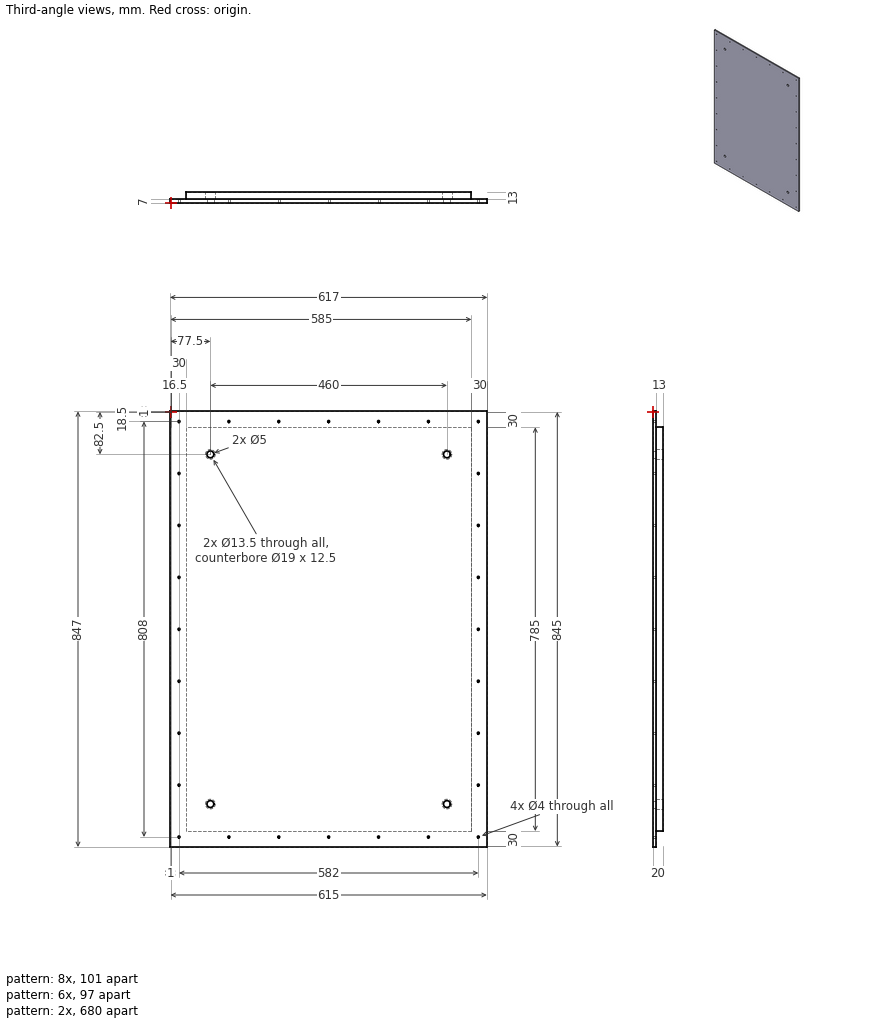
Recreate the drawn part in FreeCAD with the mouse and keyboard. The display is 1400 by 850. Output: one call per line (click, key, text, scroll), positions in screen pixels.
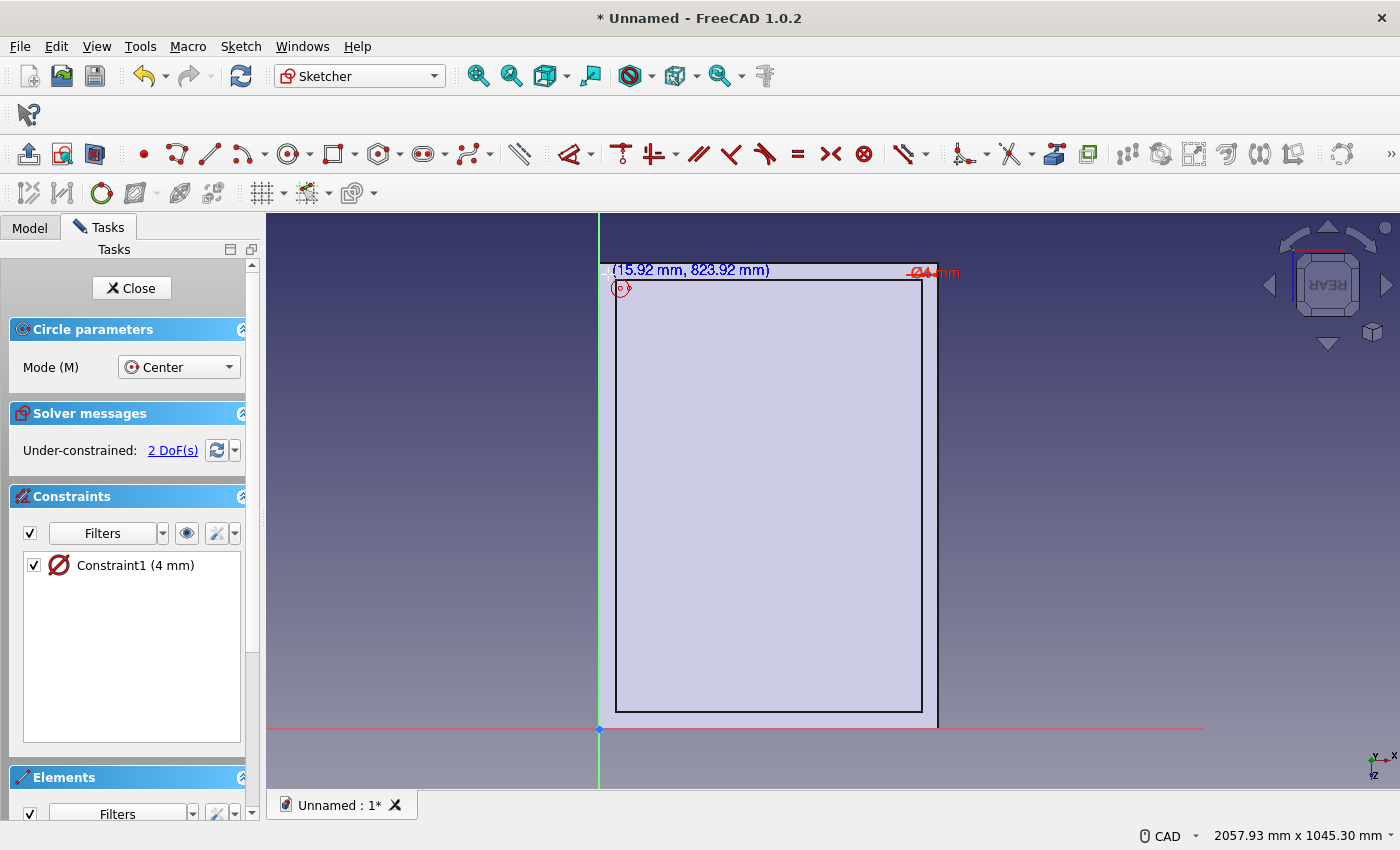
scroll(608, 274, up, 3)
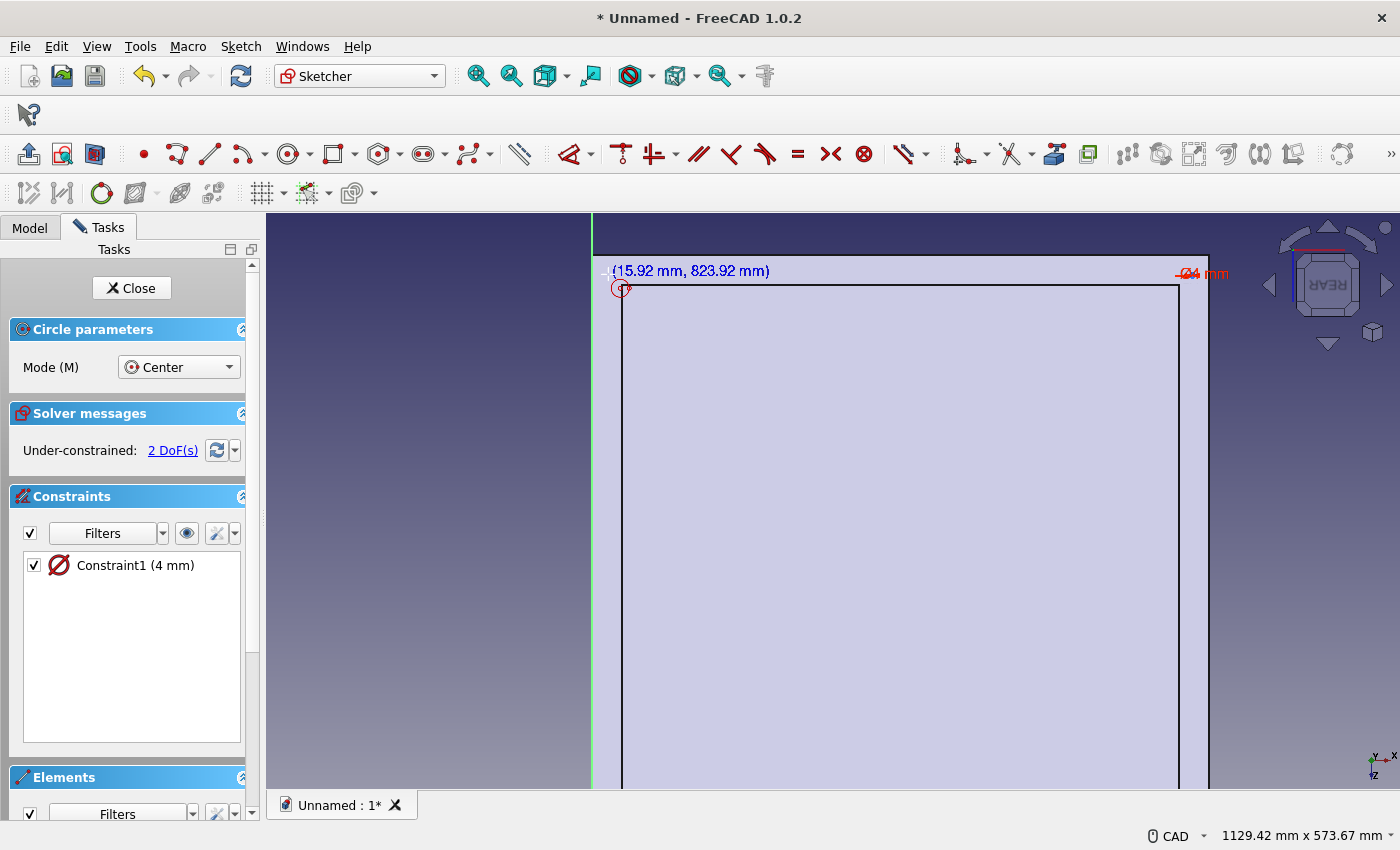
click(608, 273)
move(610, 272)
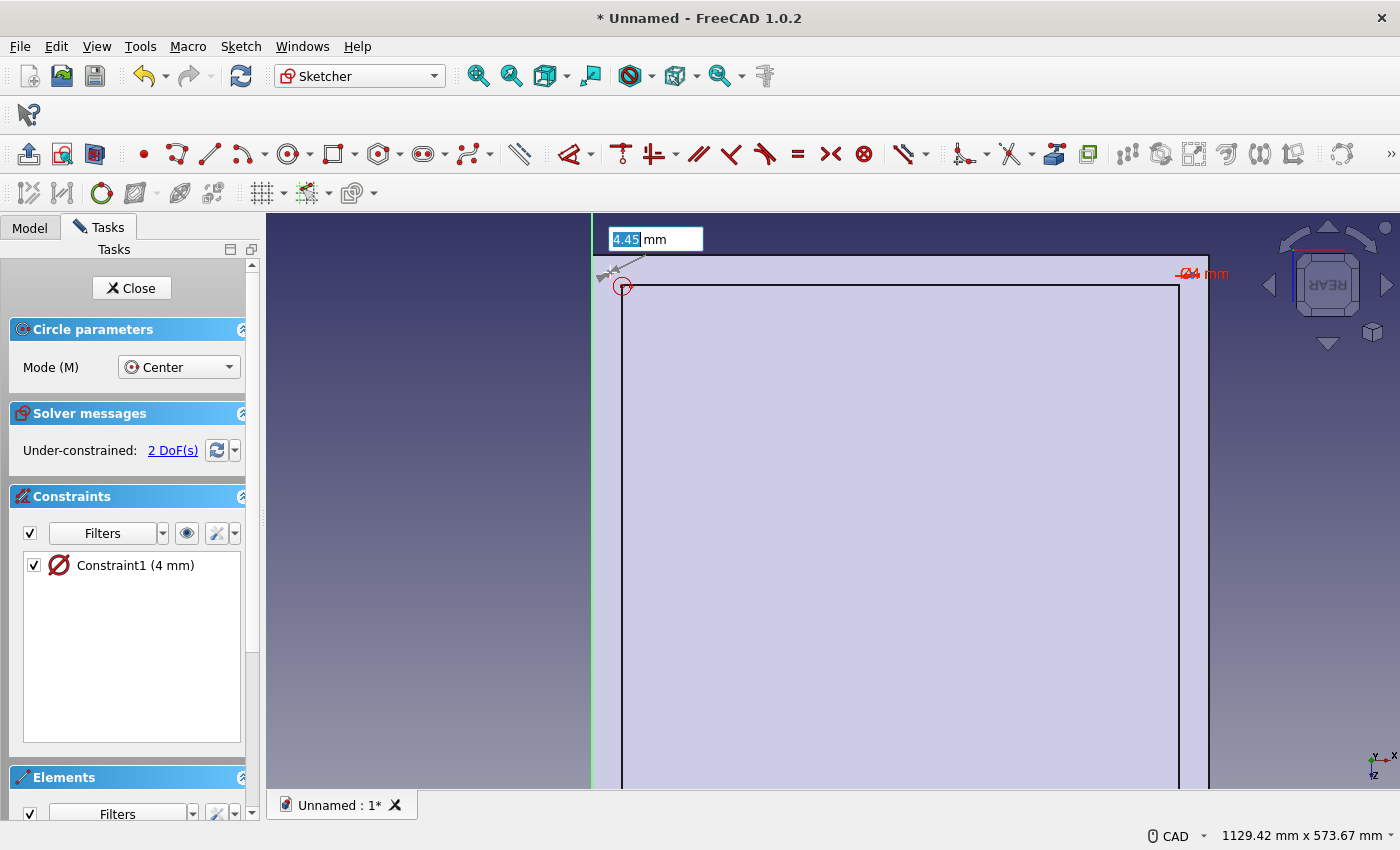
text(4)
key(Return)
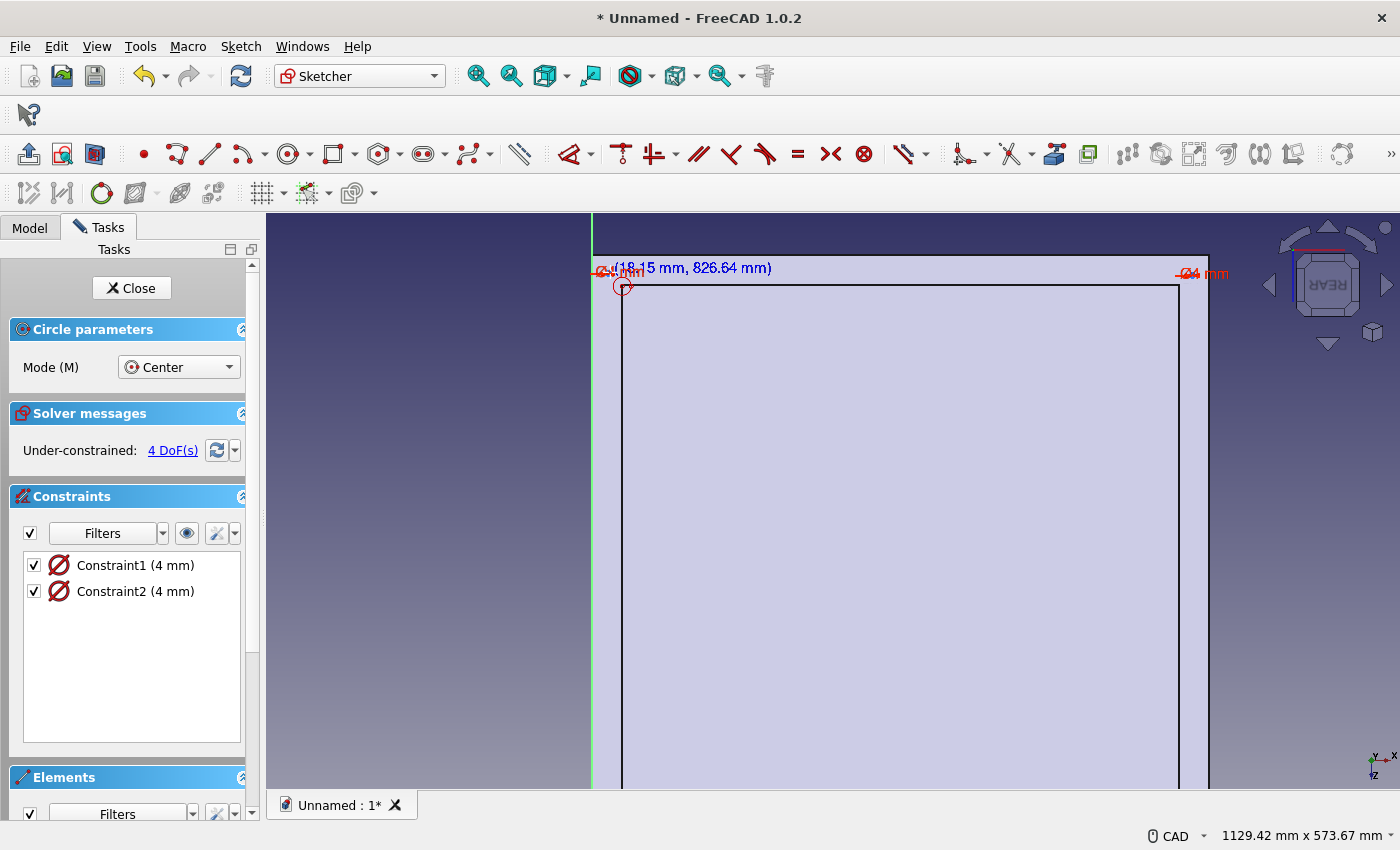
scroll(659, 349, down, 4)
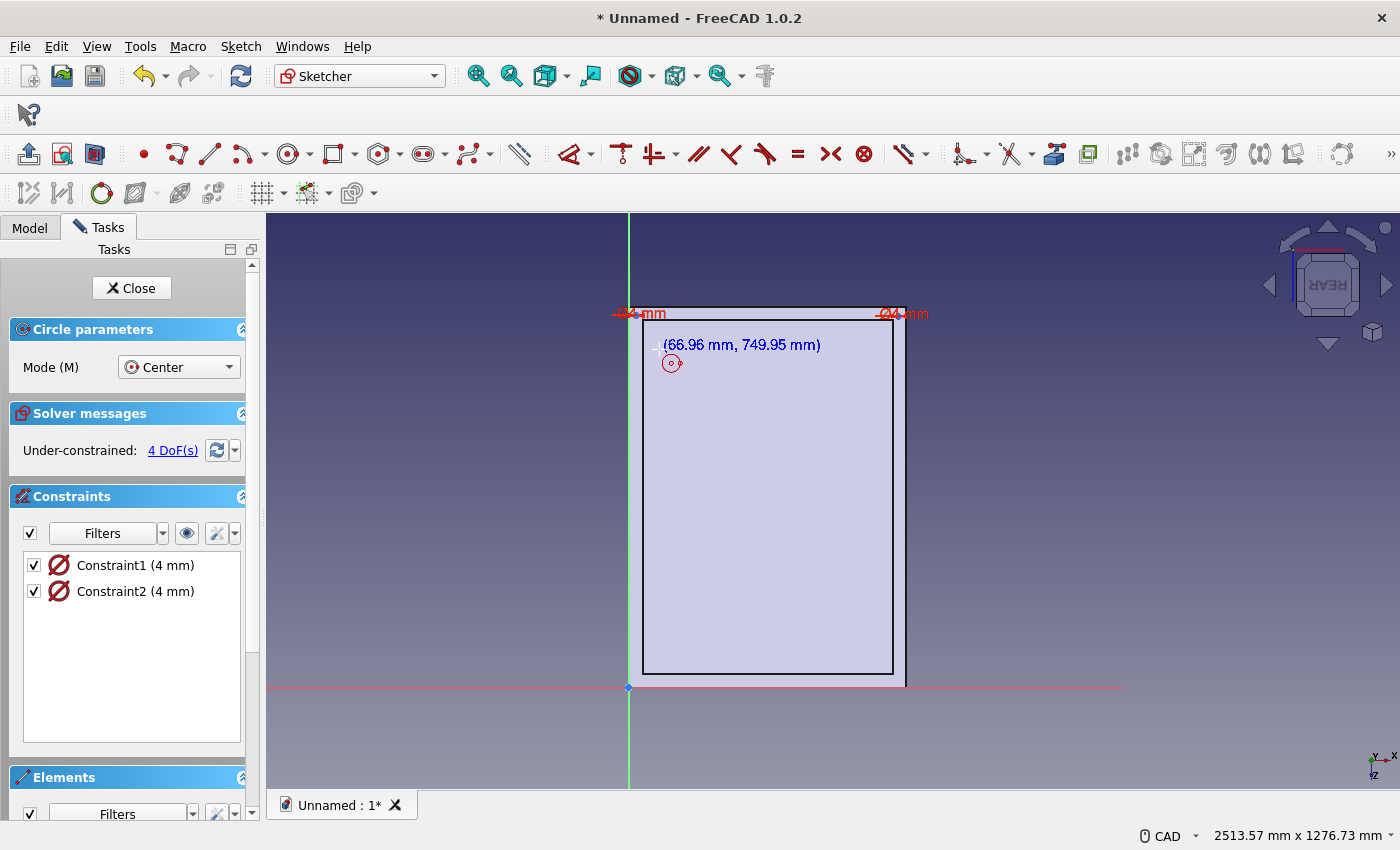
scroll(636, 680, up, 17)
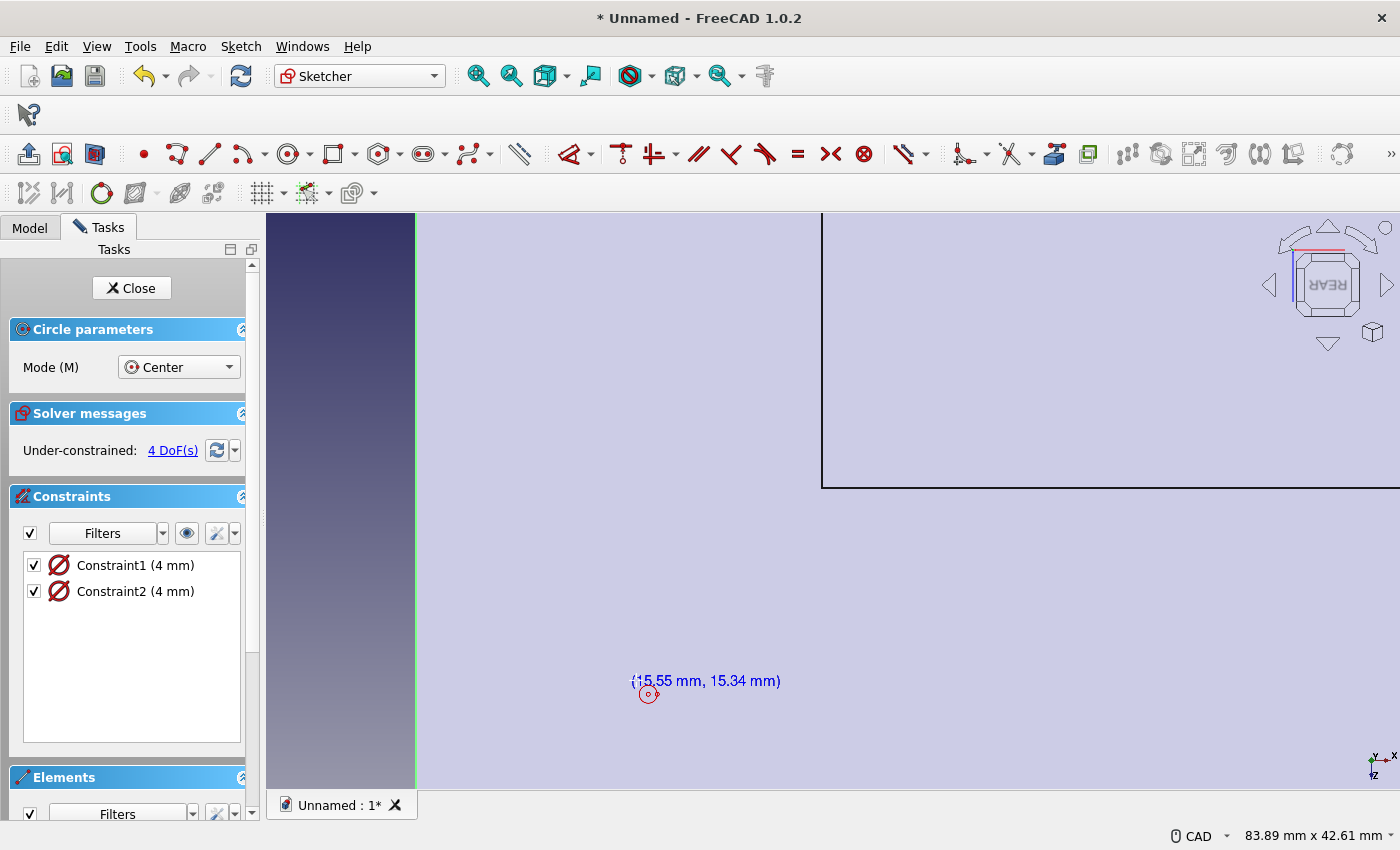
scroll(607, 722, down, 16)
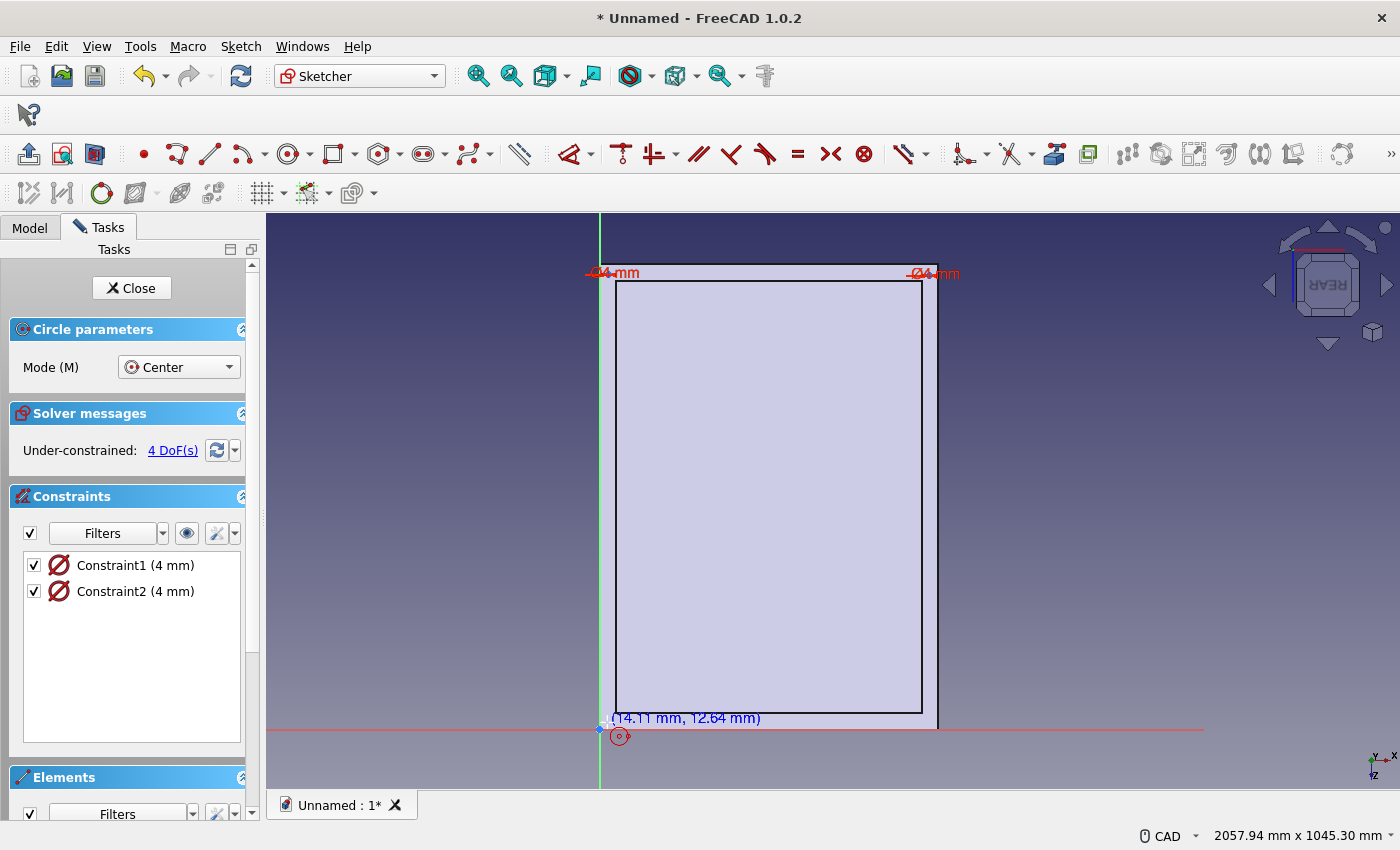
scroll(609, 720, up, 3)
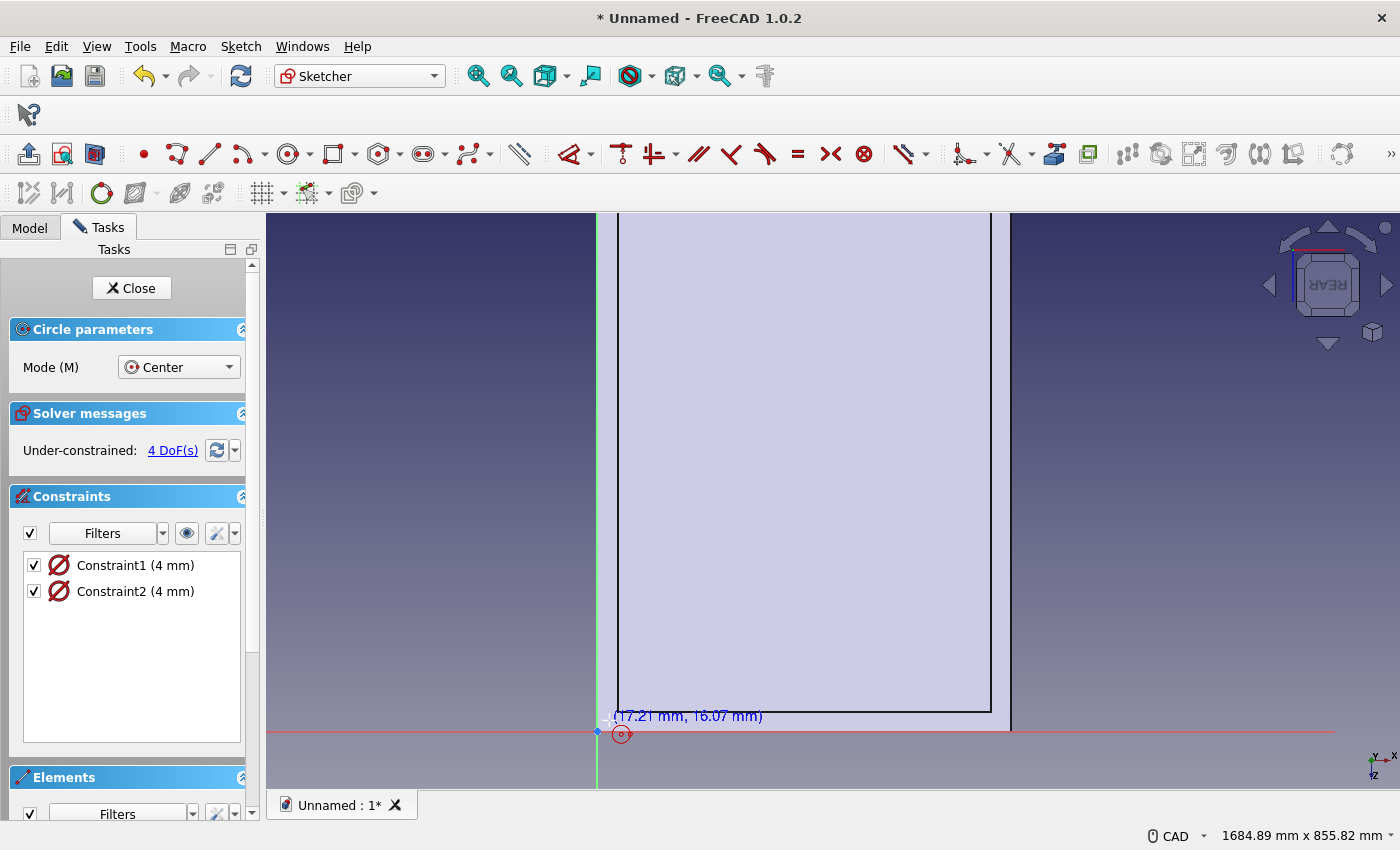
click(608, 719)
move(609, 717)